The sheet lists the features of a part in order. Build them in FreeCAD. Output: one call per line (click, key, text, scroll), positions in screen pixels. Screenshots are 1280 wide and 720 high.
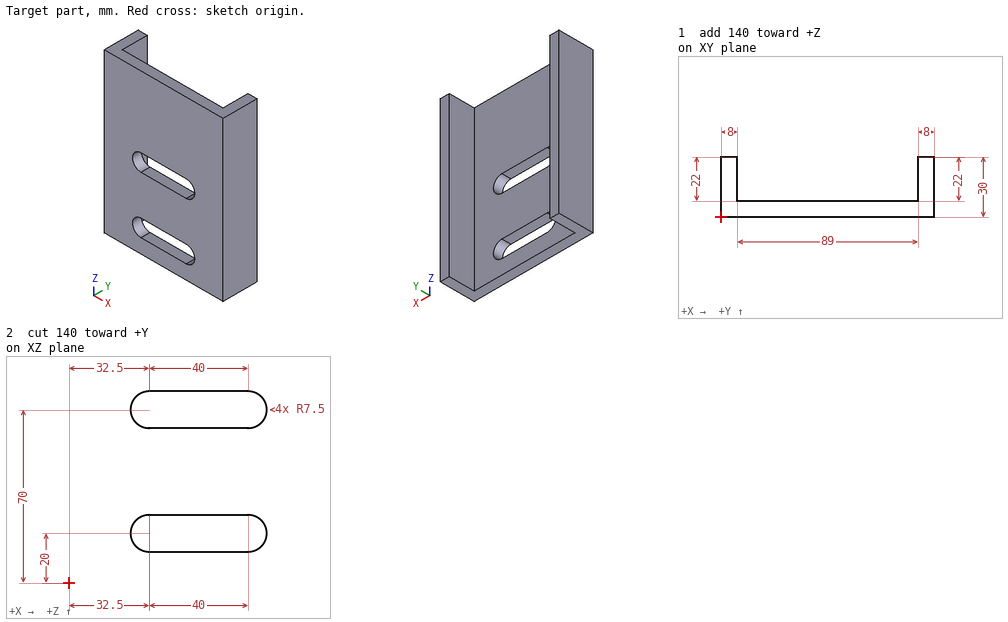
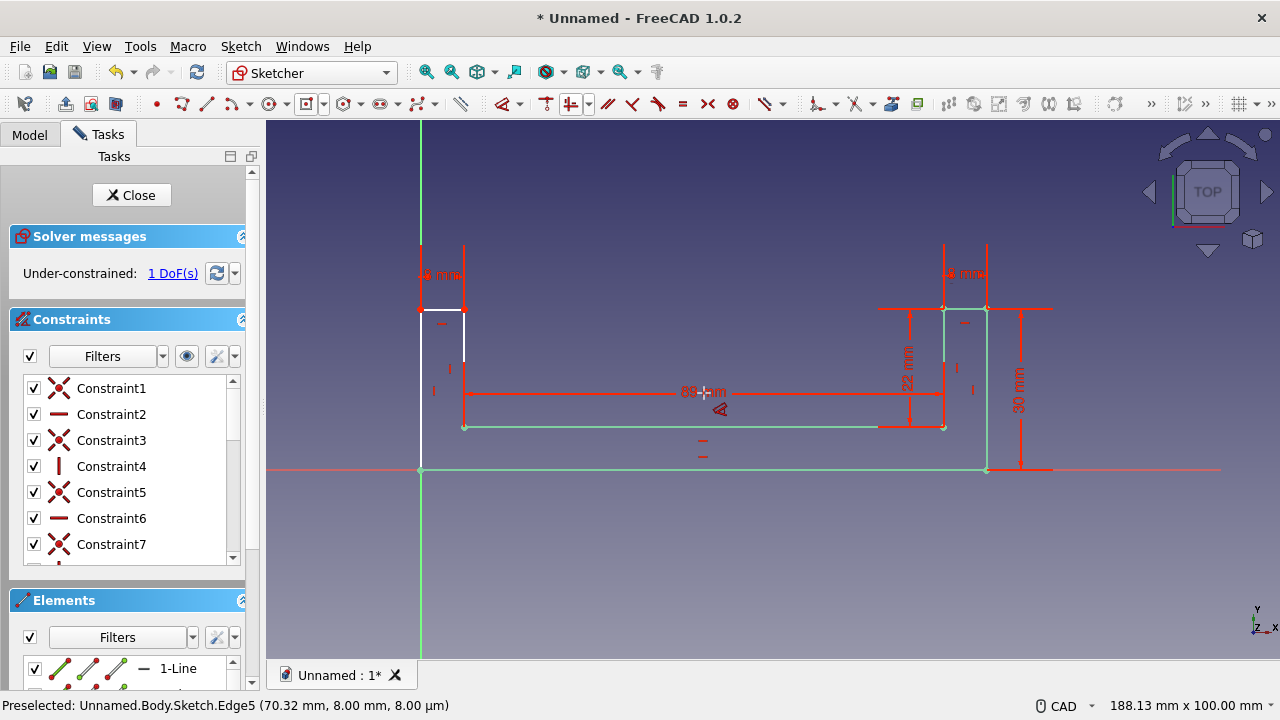
click(464, 392)
click(498, 369)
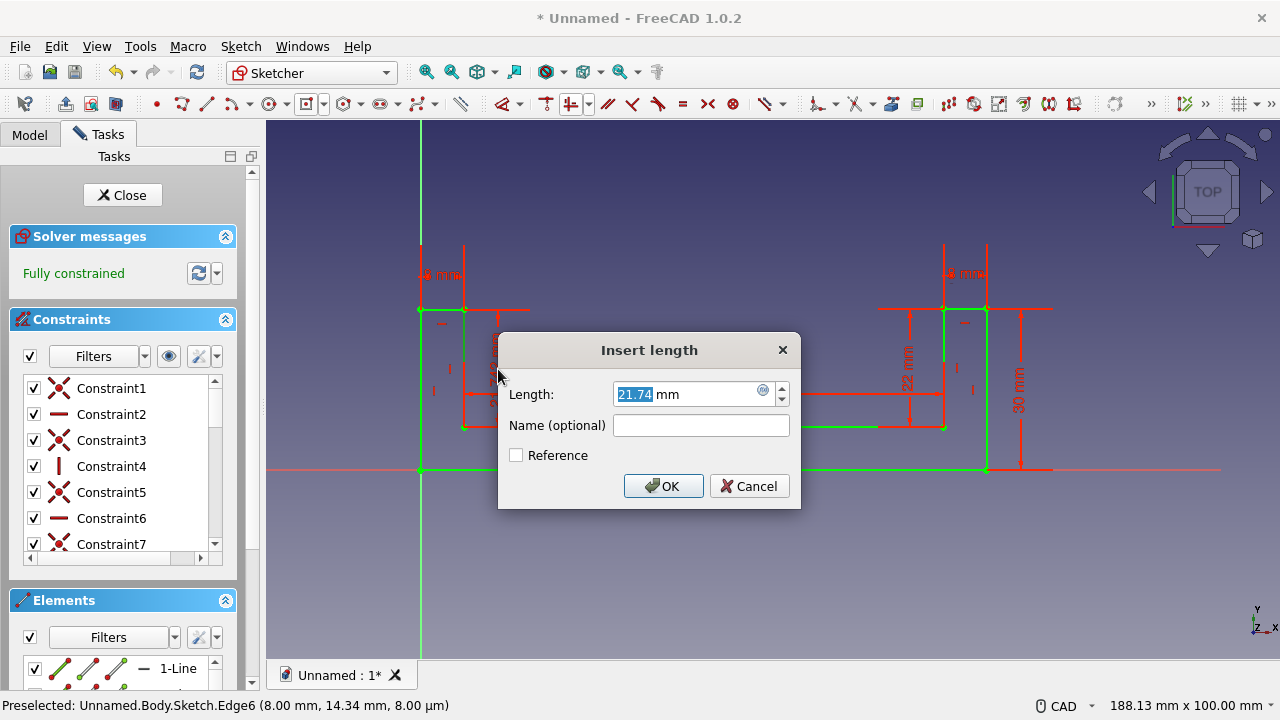
text(22)
key(Return)
key(Escape)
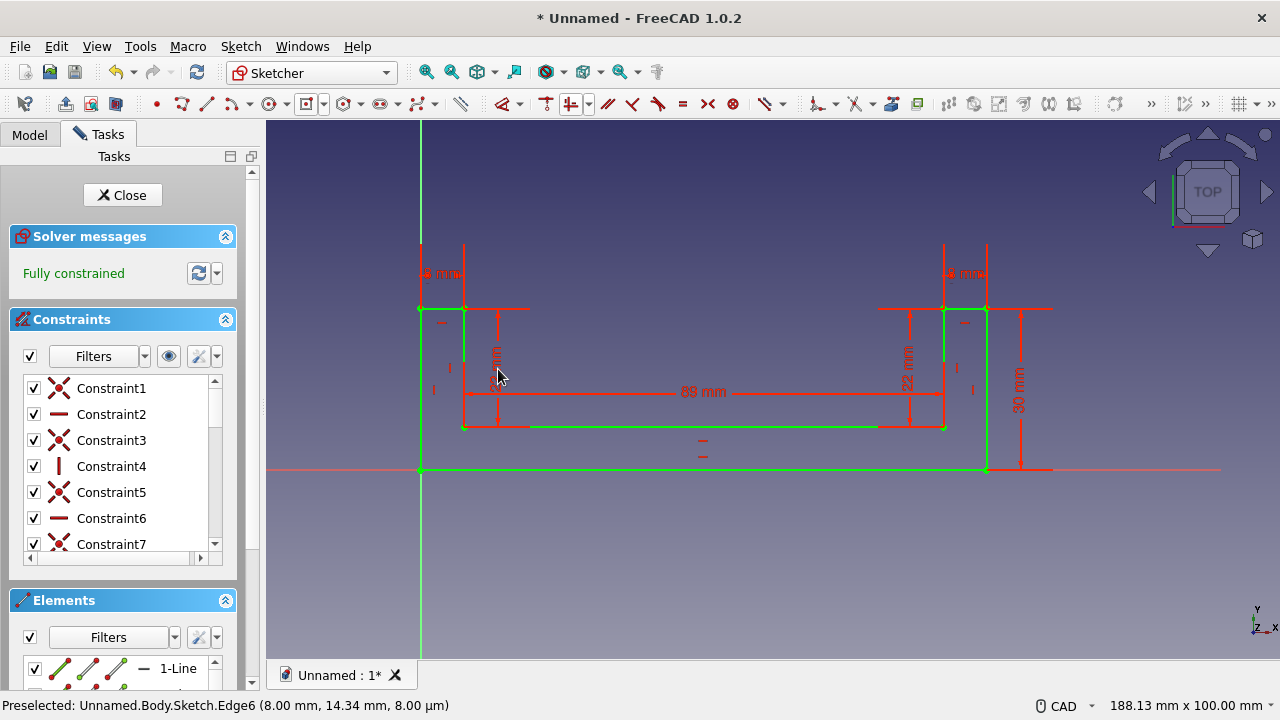
click(123, 195)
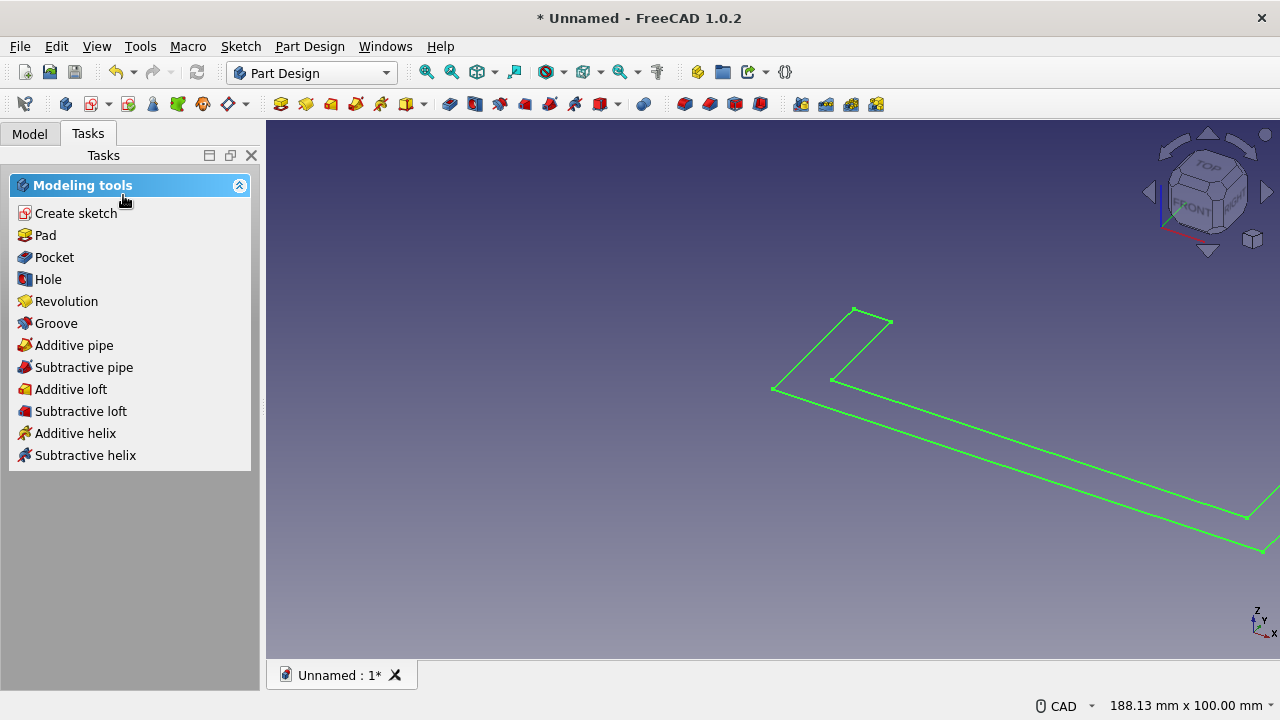
click(281, 104)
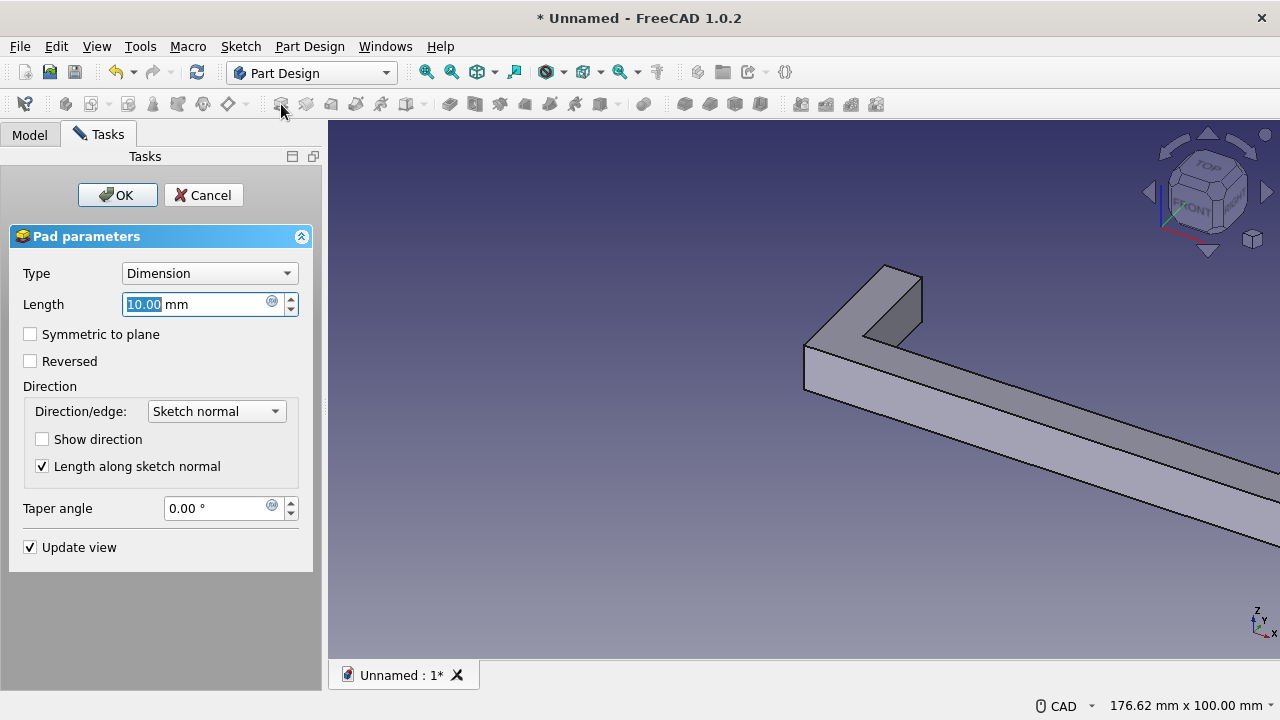
text(140)
key(Tab)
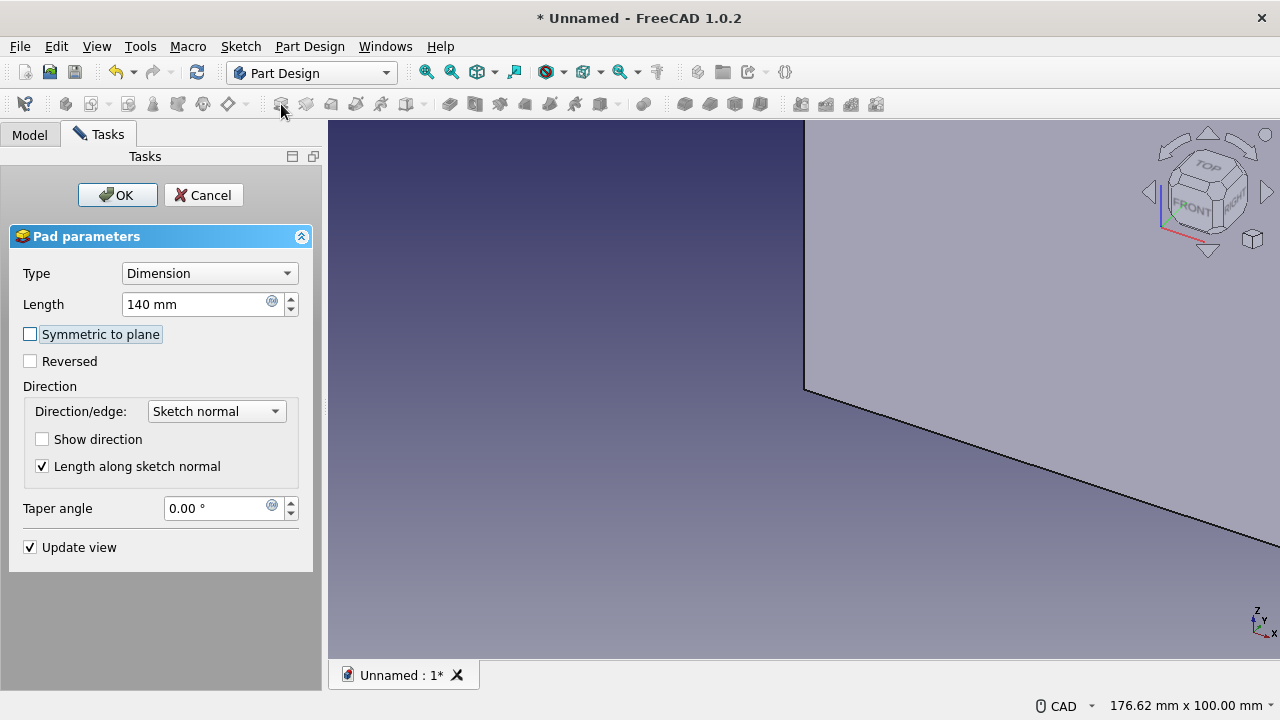
click(118, 195)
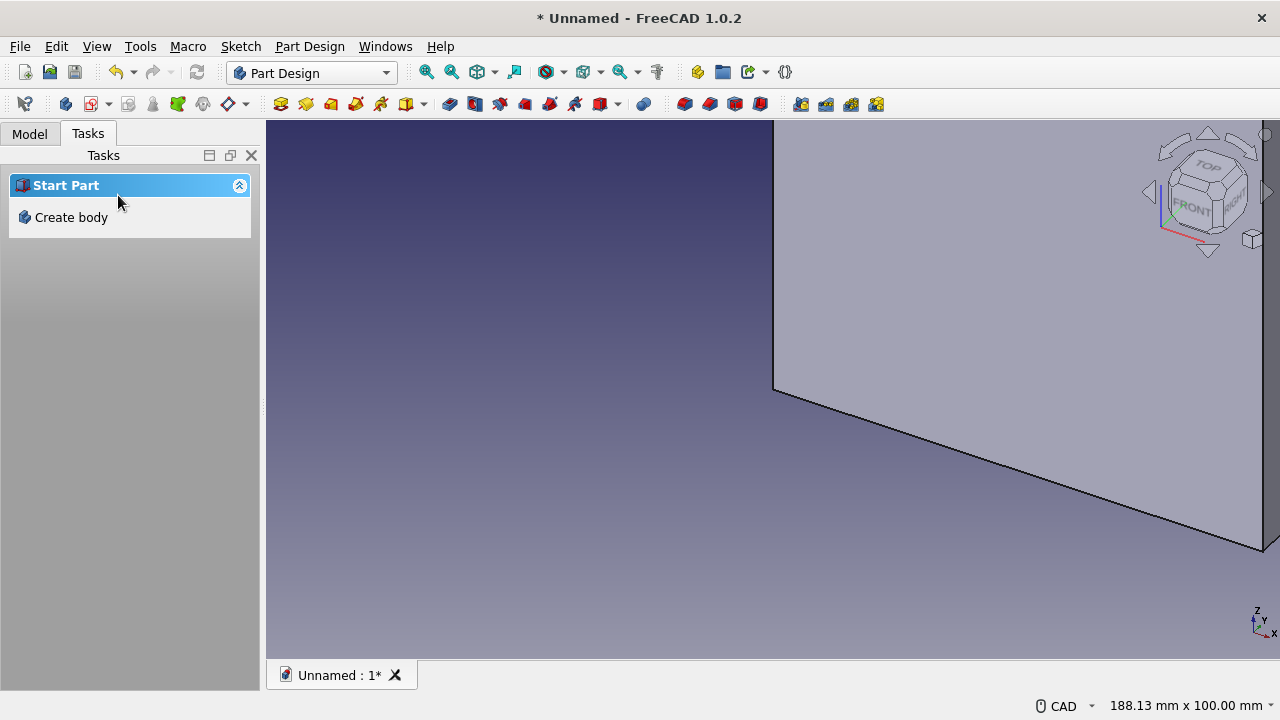
click(427, 72)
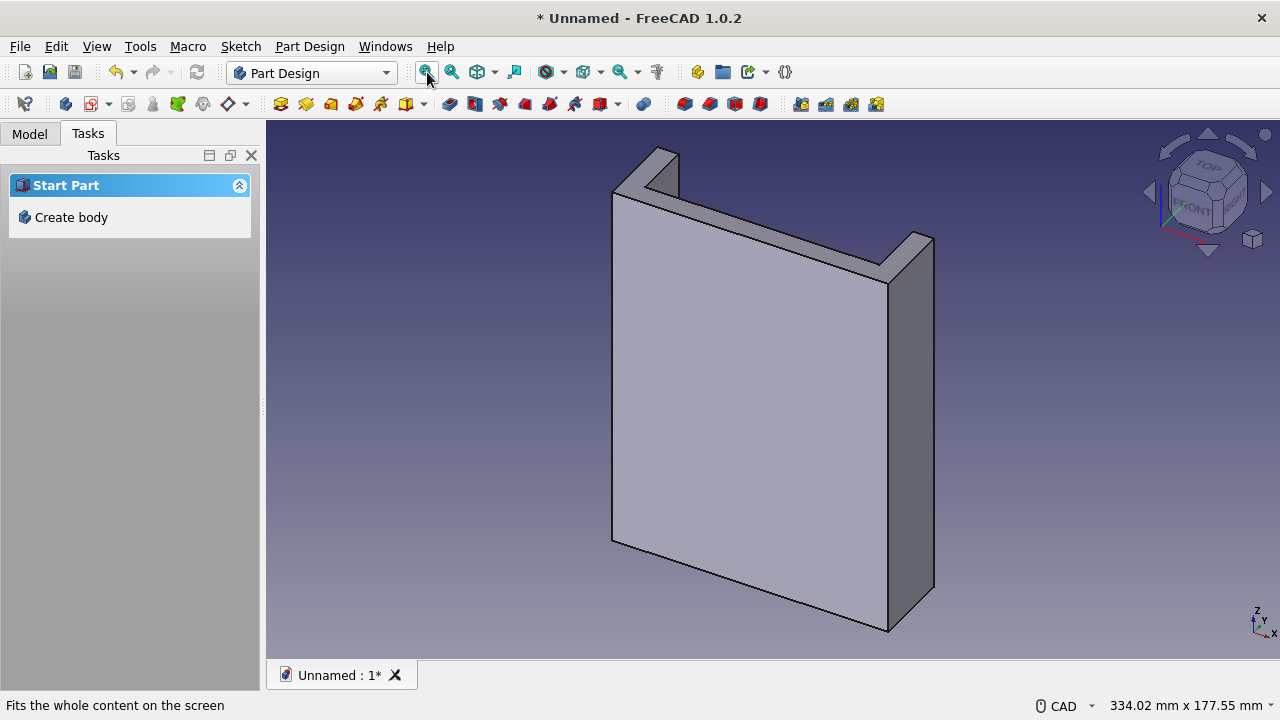
click(90, 104)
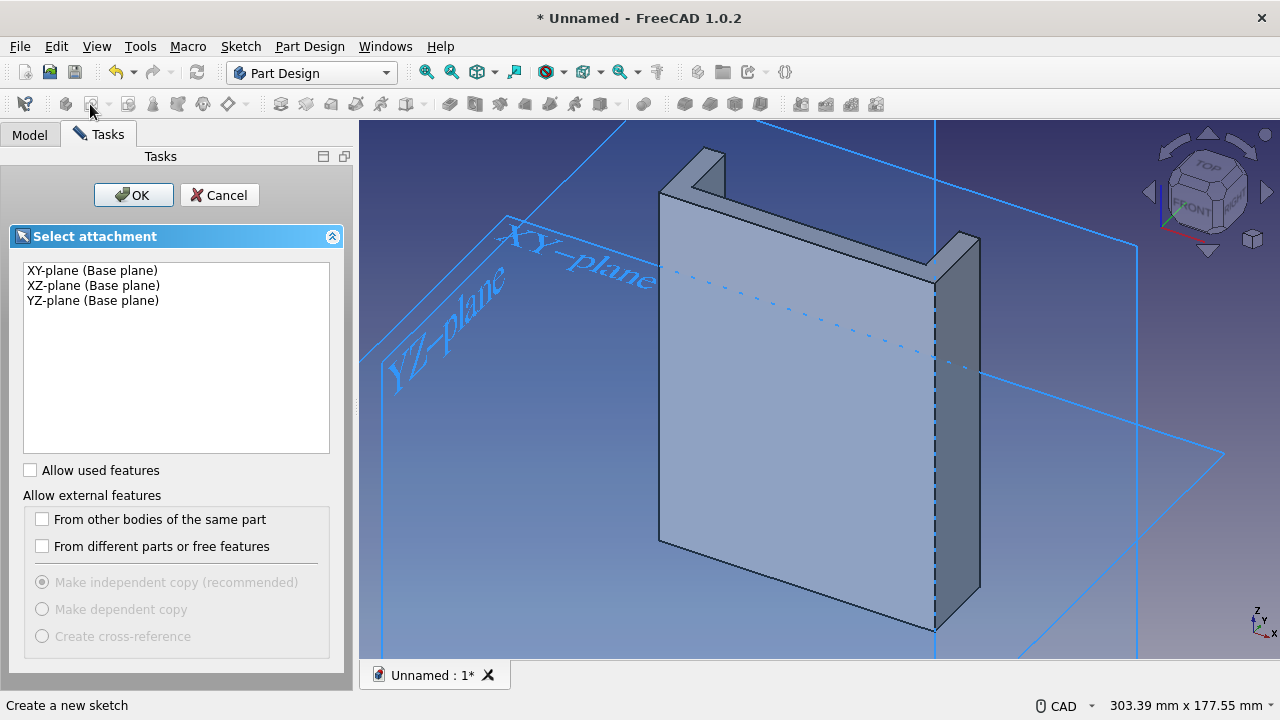
click(84, 286)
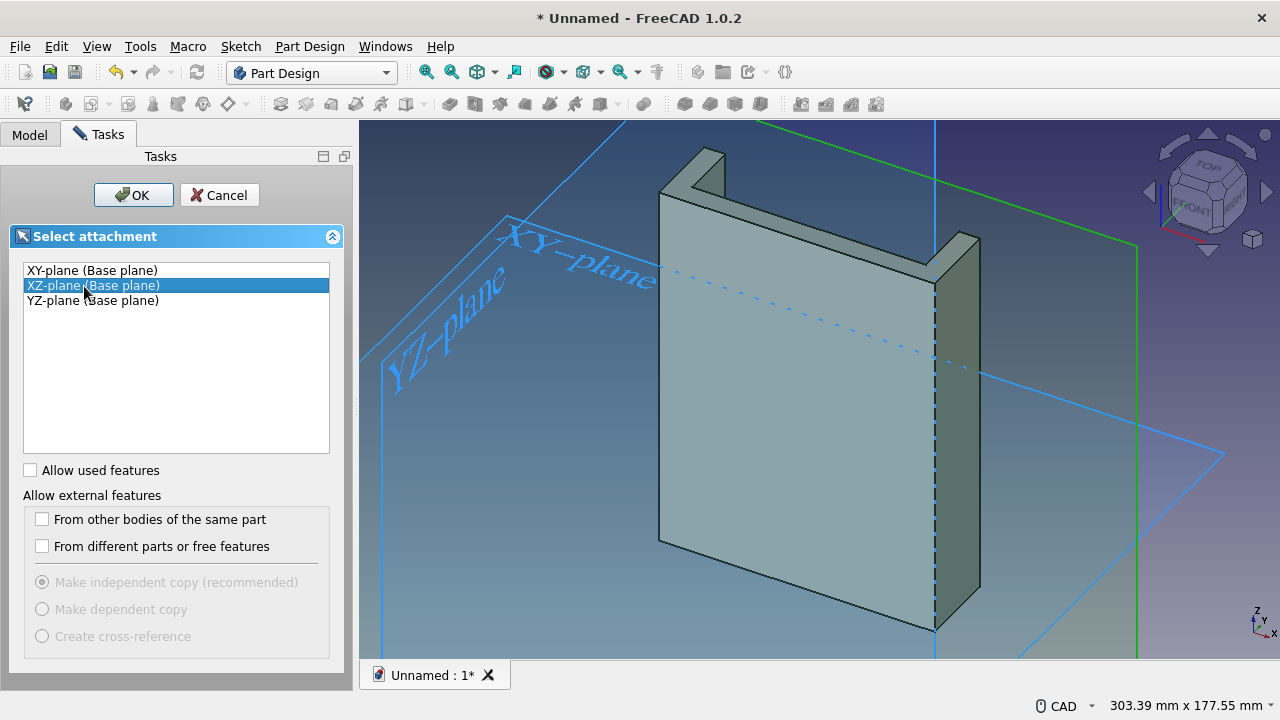
click(134, 195)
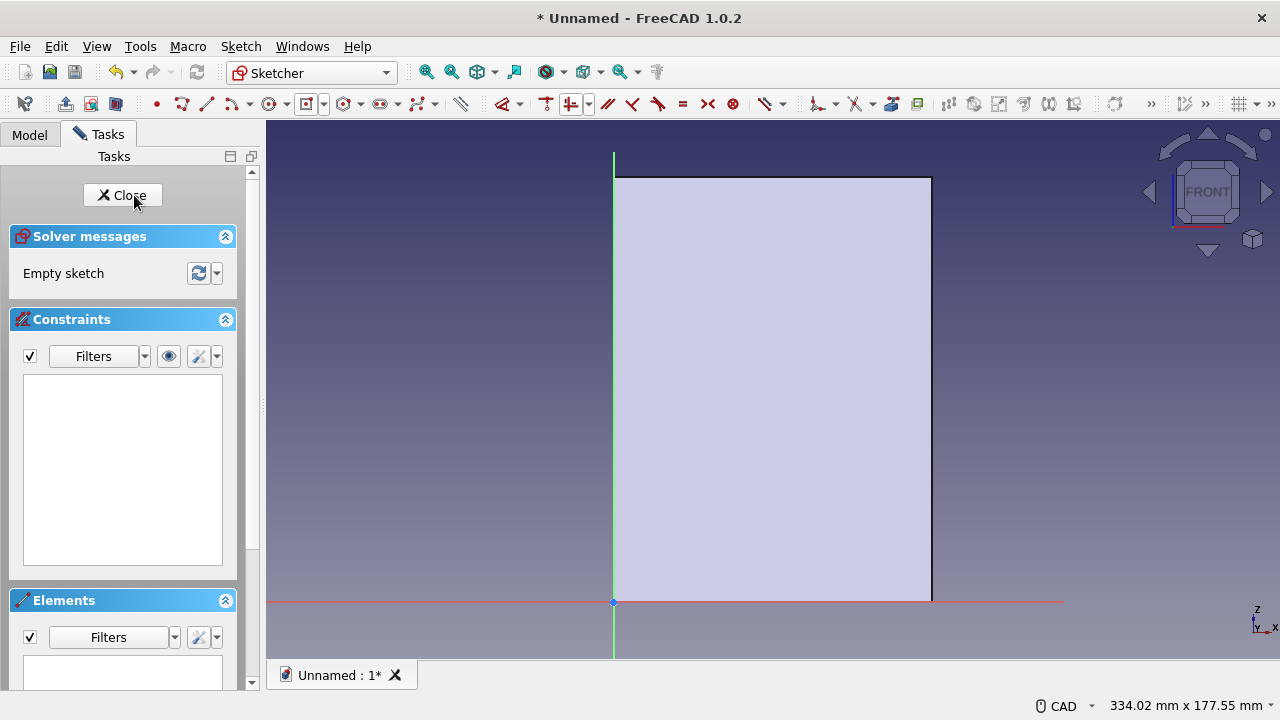
scroll(797, 631, up, 2)